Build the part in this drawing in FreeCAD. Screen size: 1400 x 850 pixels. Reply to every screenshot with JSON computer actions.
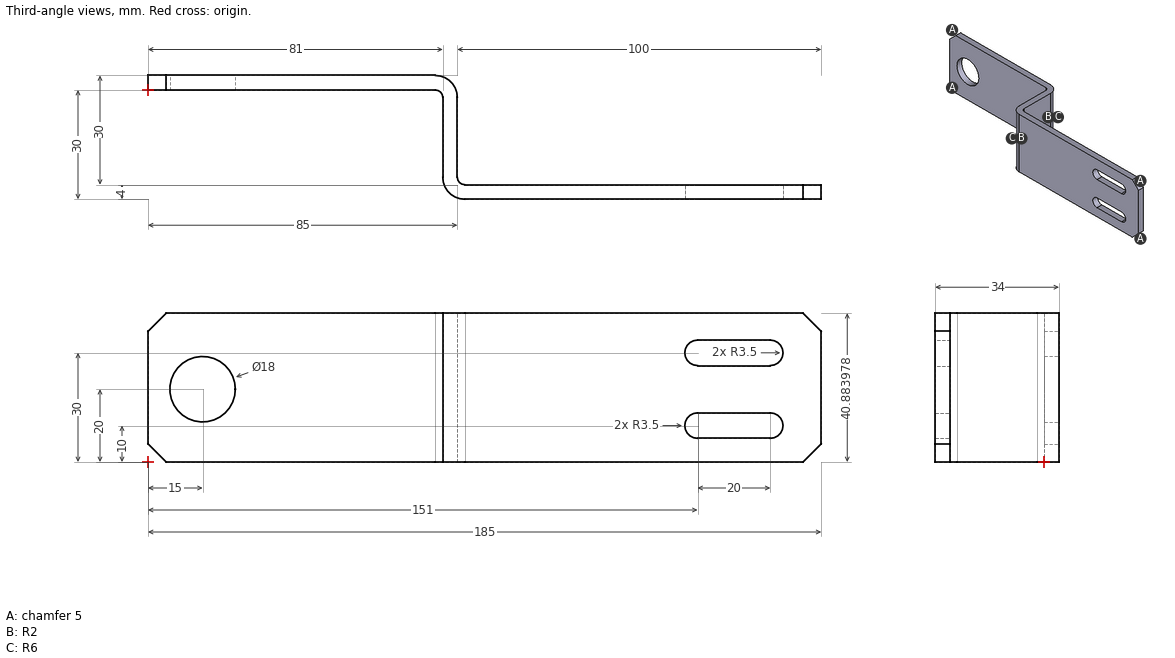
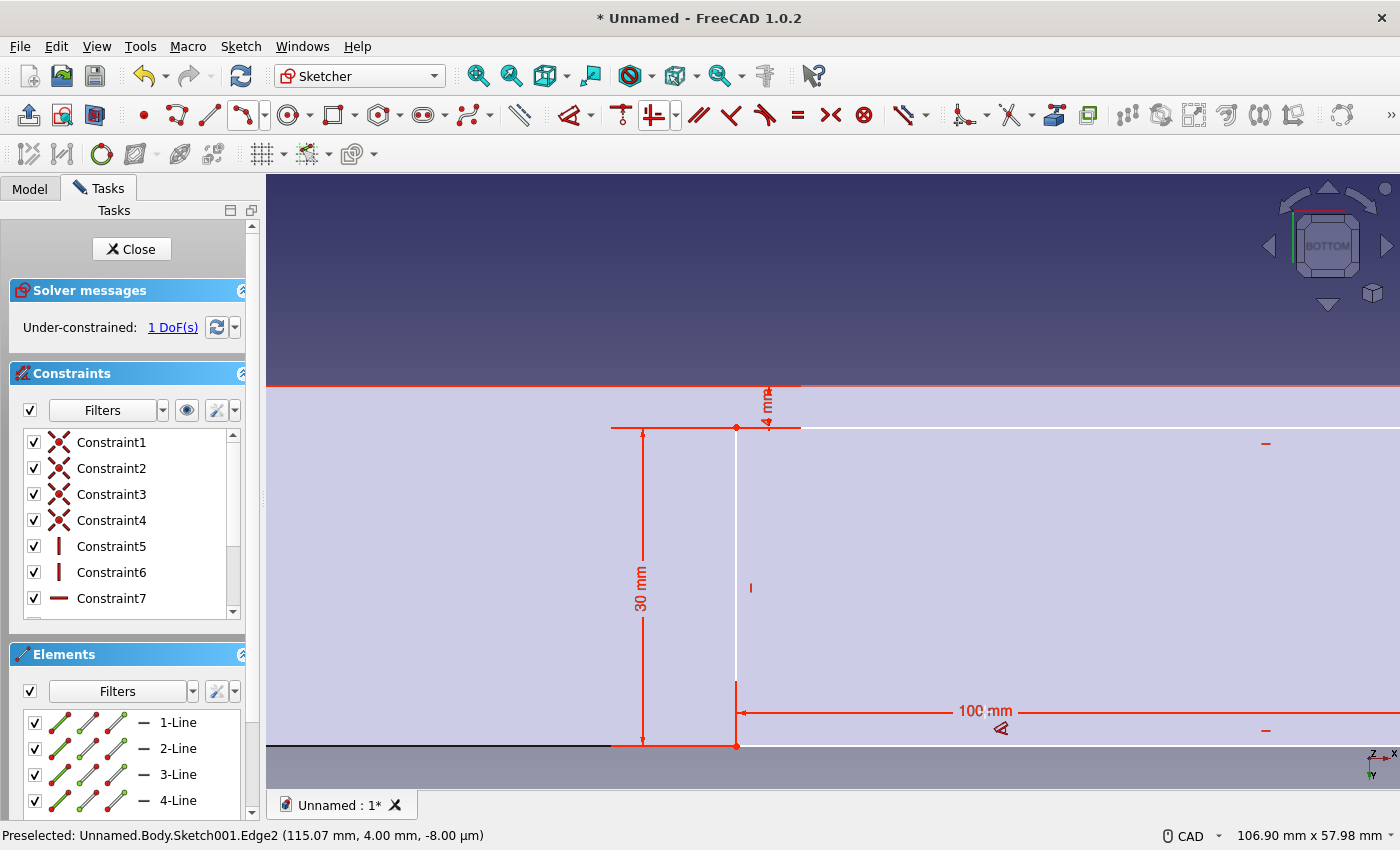
{"action": "left_click", "coordinate": [736, 428]}
{"action": "left_click", "coordinate": [515, 352]}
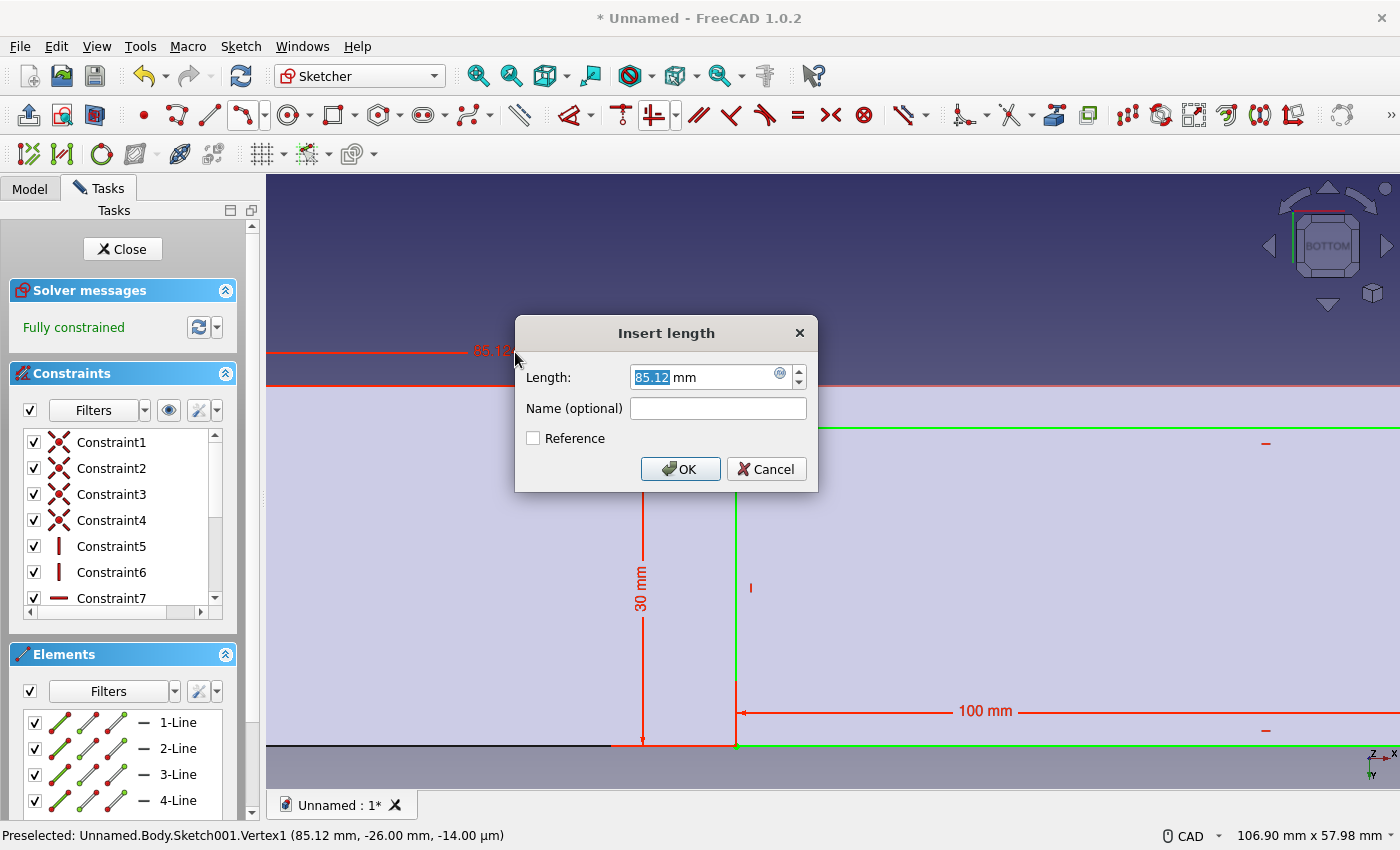
{"action": "type", "text": "85"}
{"action": "key", "text": "Return"}
{"action": "key", "text": "Escape"}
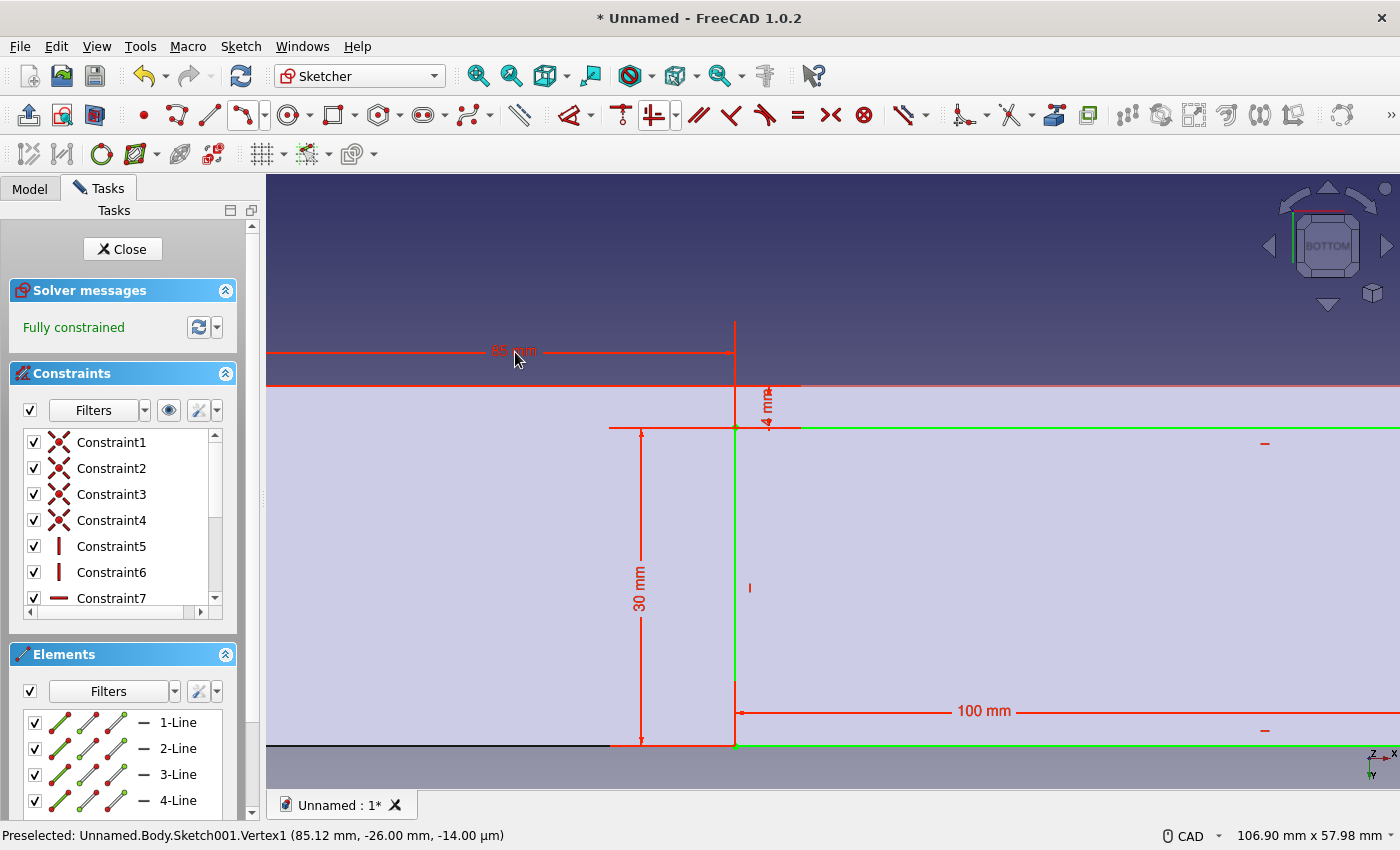
{"action": "left_click", "coordinate": [123, 249]}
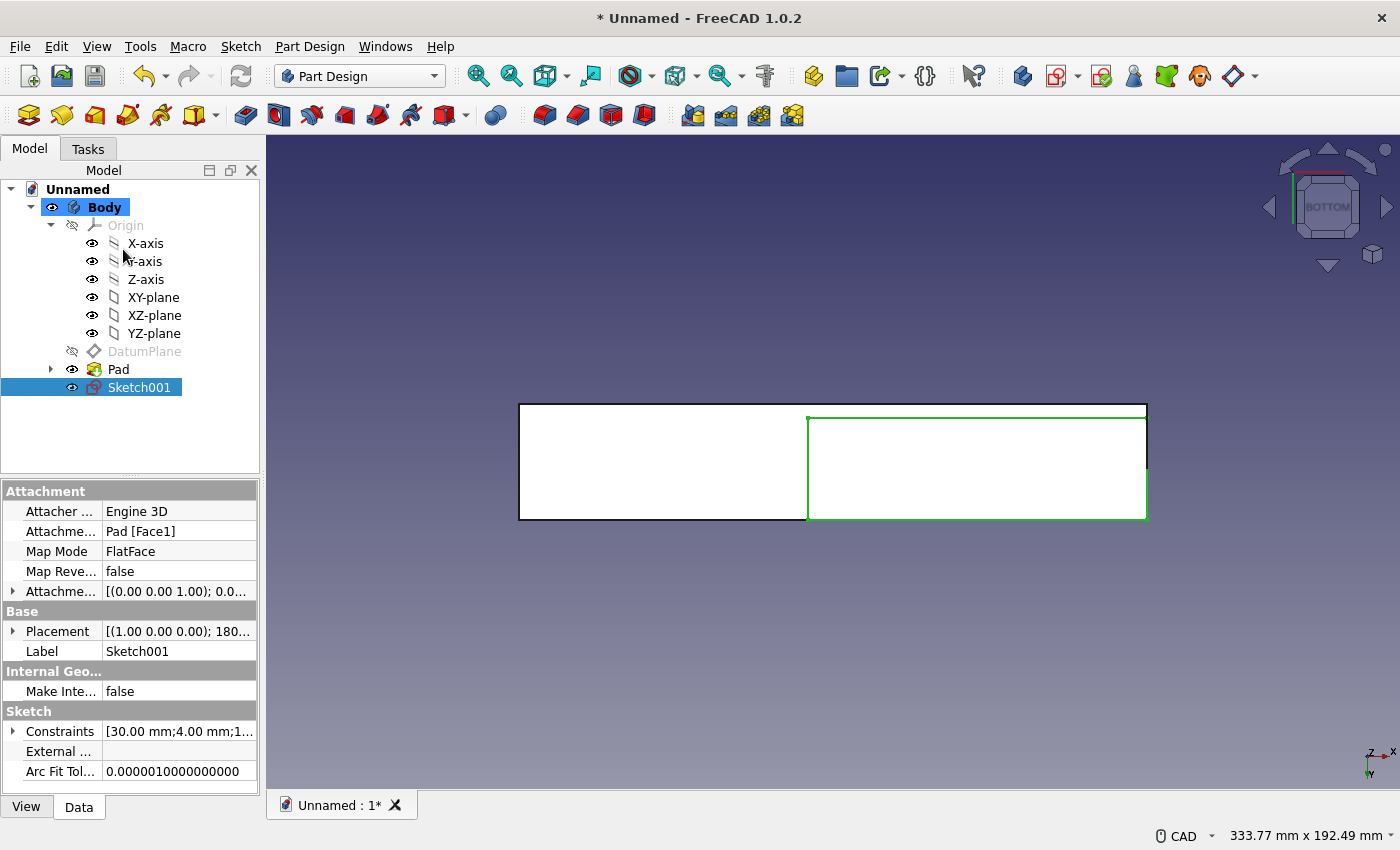
{"action": "left_click", "coordinate": [246, 116]}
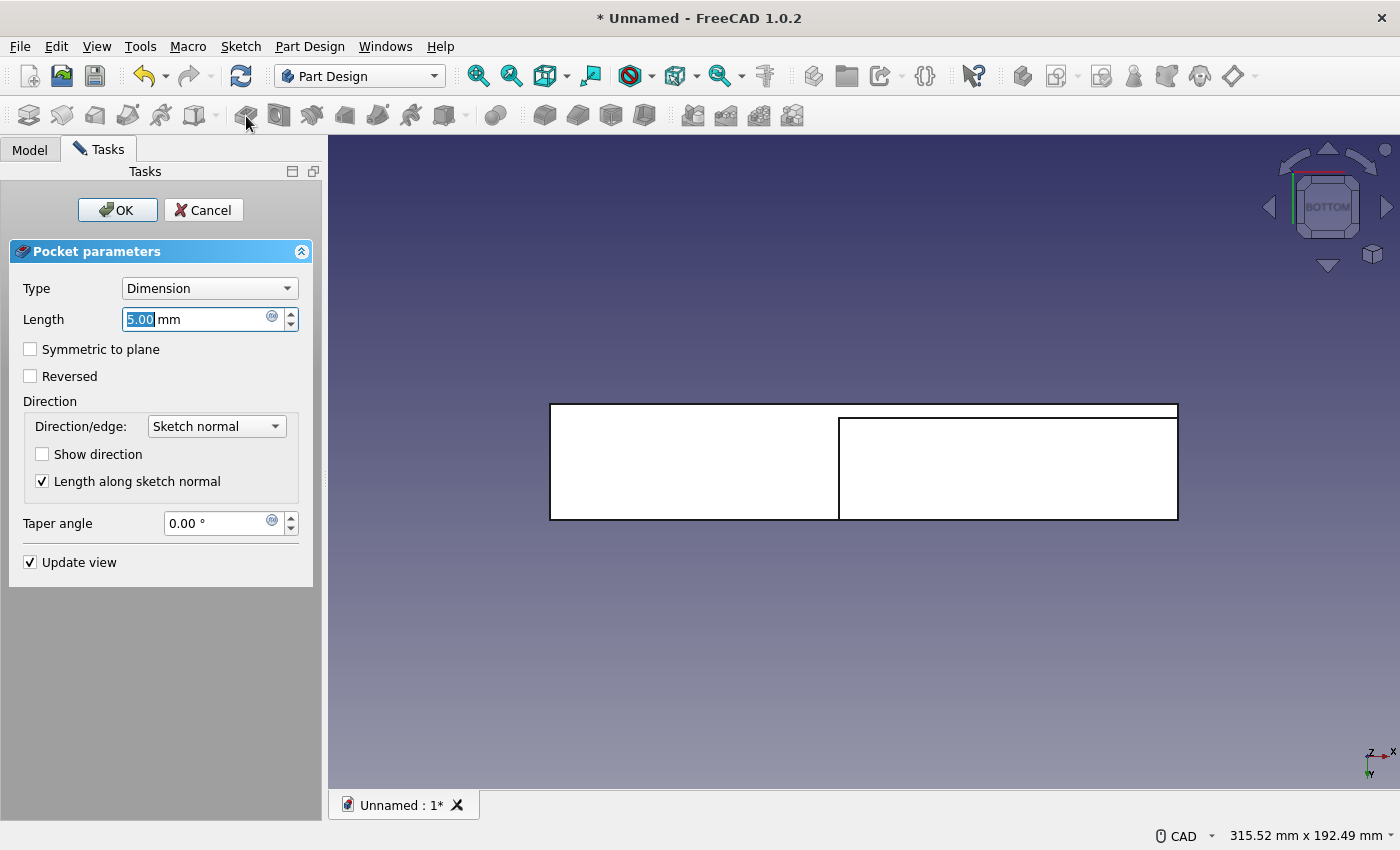
{"action": "left_click", "coordinate": [210, 288]}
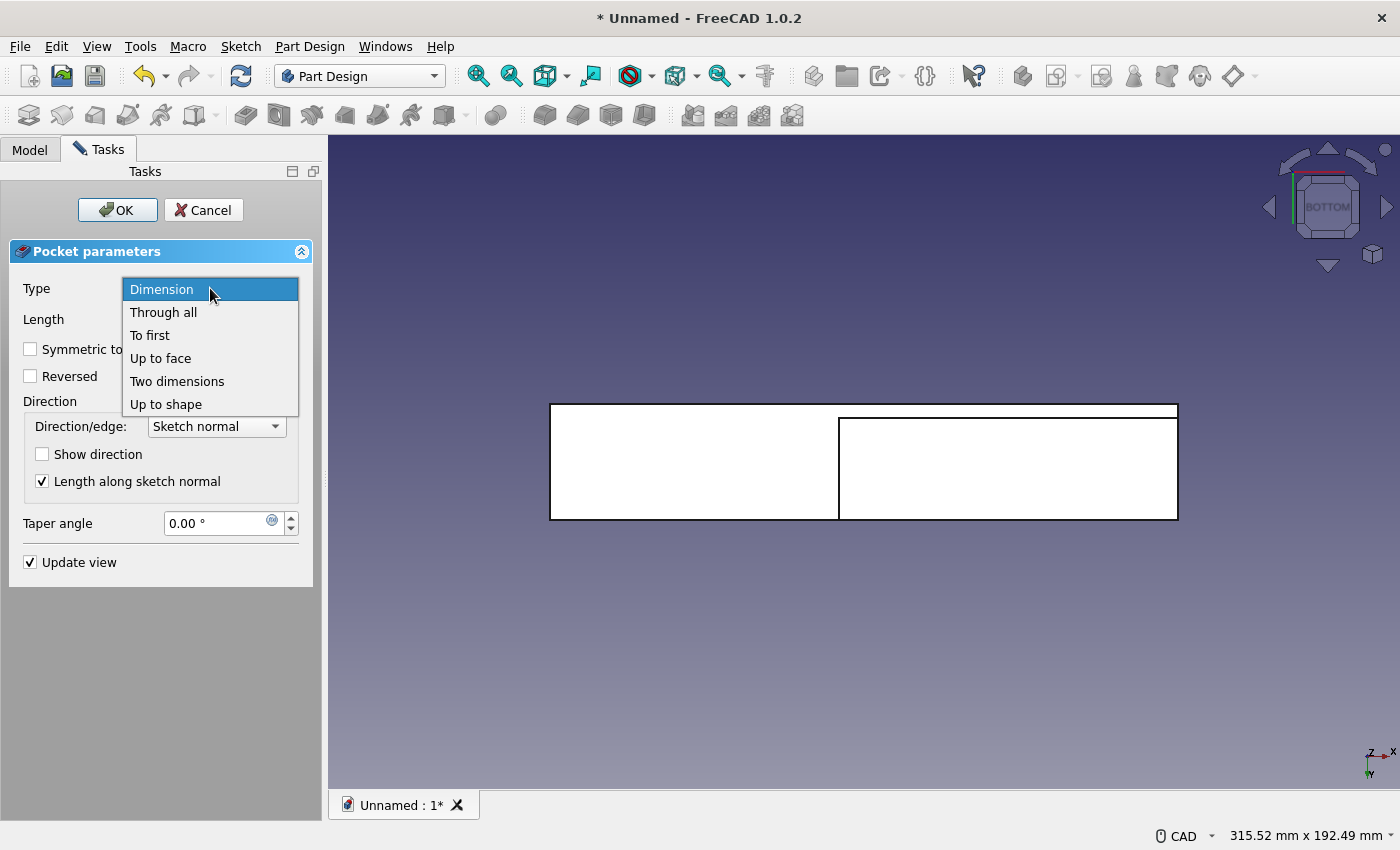
{"action": "left_click", "coordinate": [208, 312]}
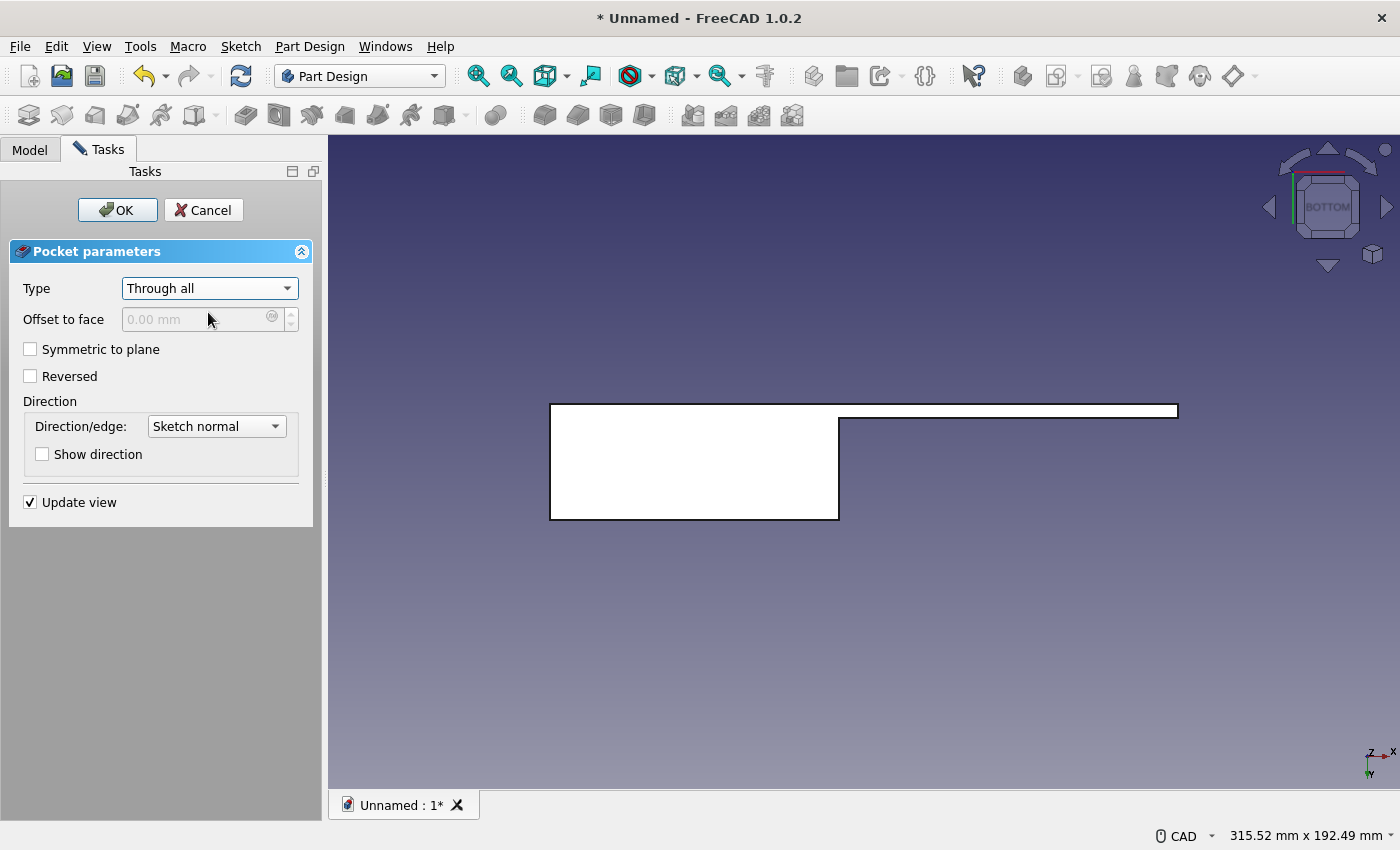
{"action": "left_click", "coordinate": [118, 210]}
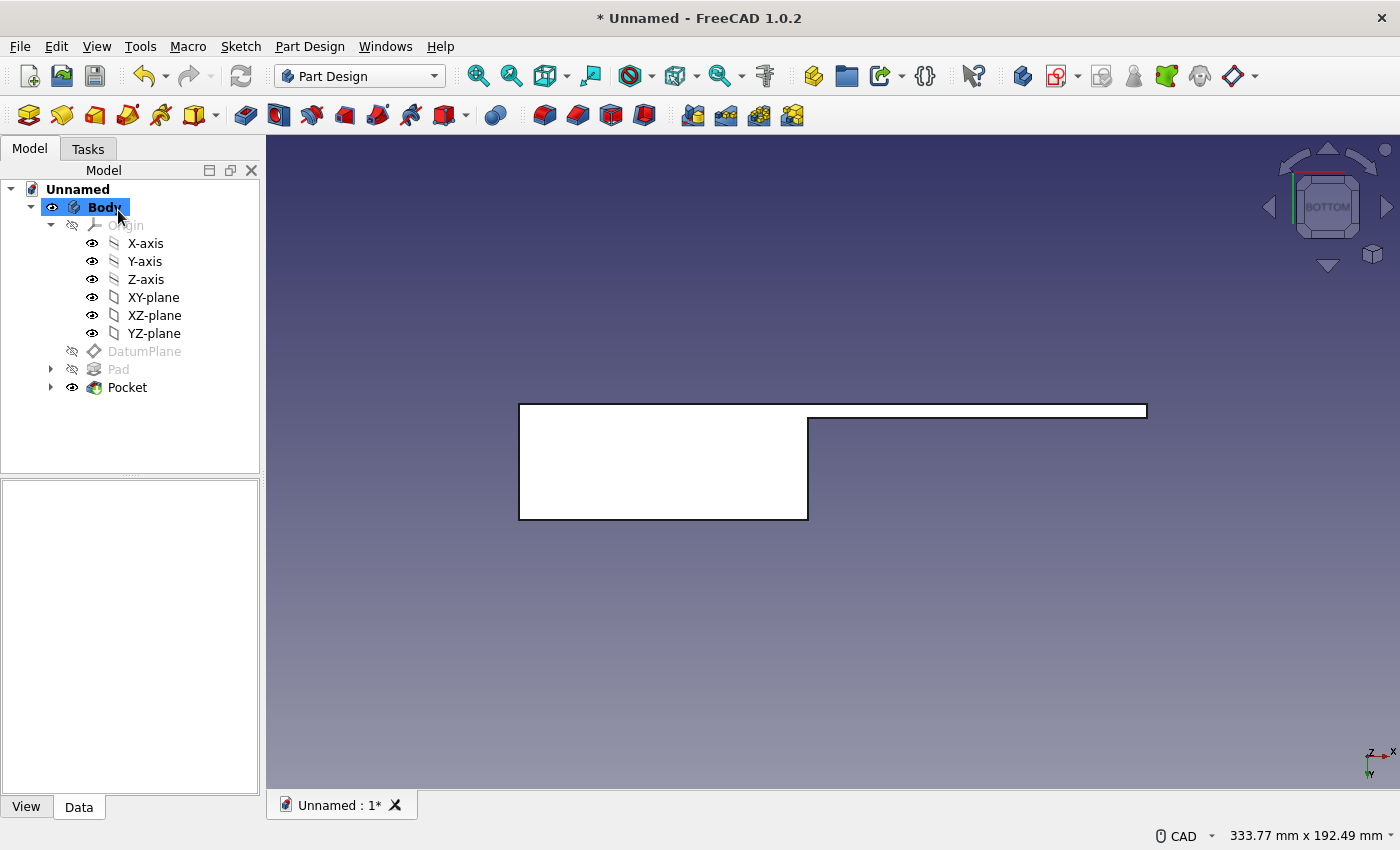
{"action": "left_click", "coordinate": [743, 461]}